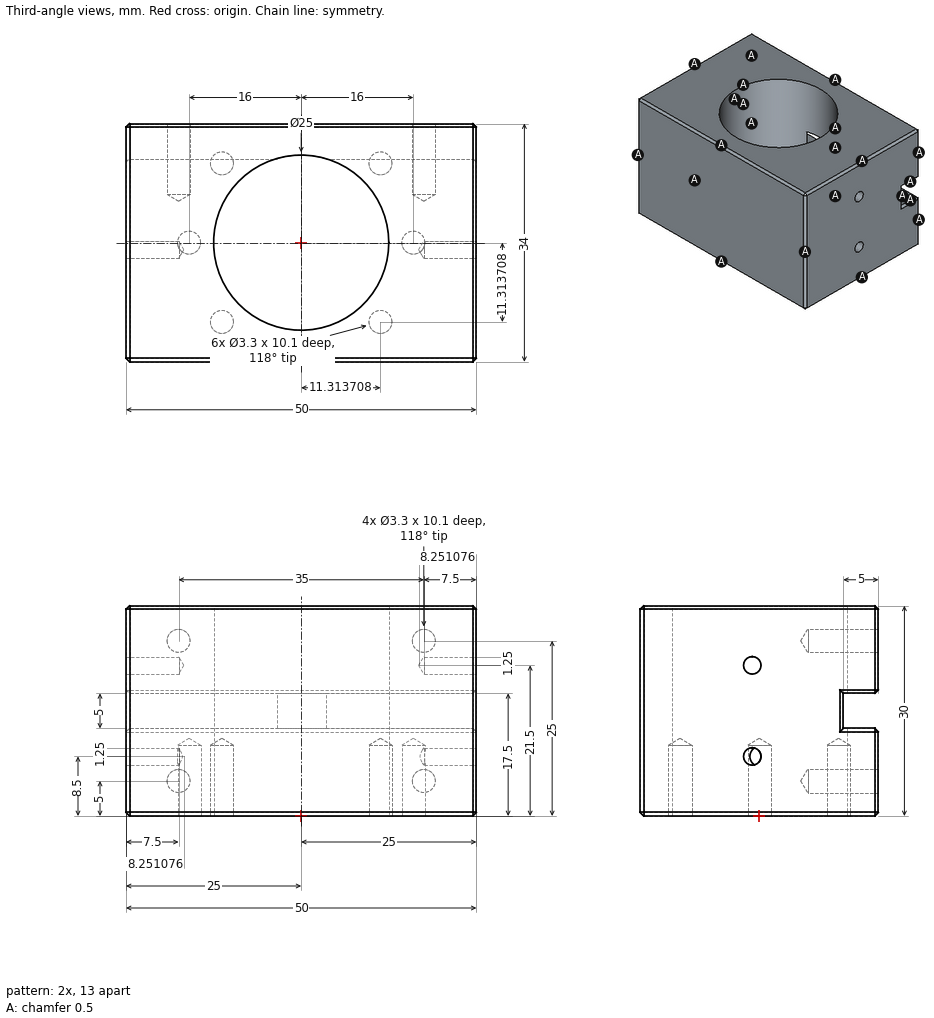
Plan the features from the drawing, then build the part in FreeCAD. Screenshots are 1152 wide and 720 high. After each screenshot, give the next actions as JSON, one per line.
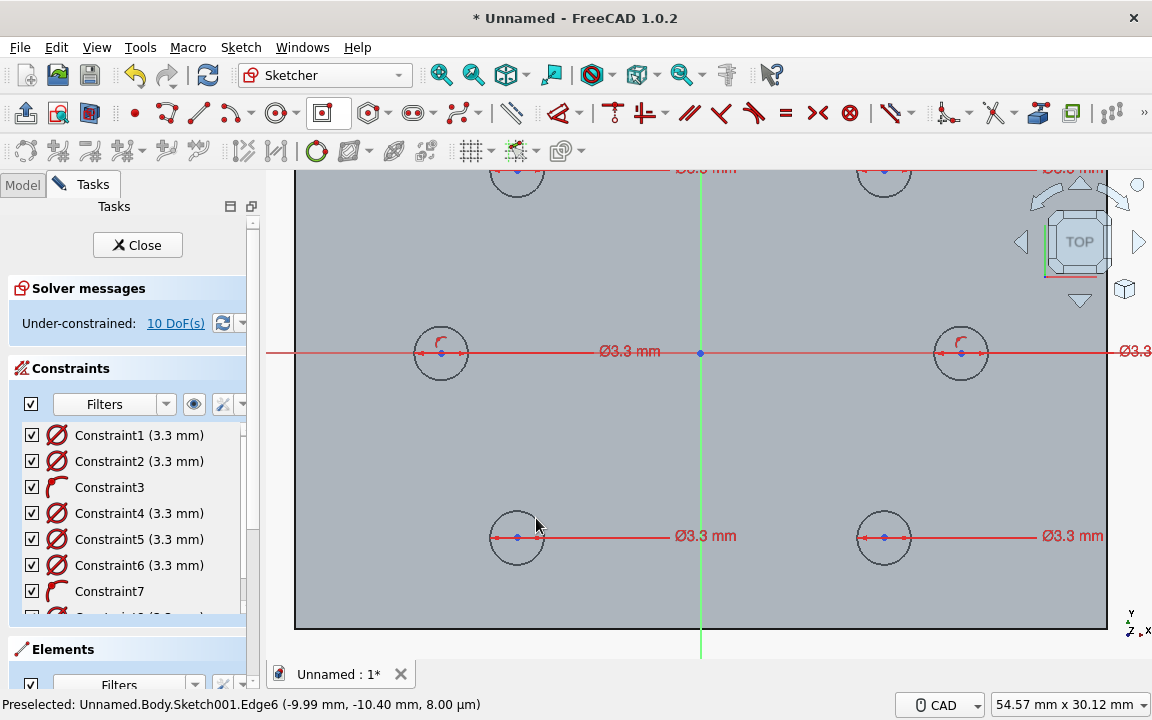
{"action": "left_click", "coordinate": [884, 538]}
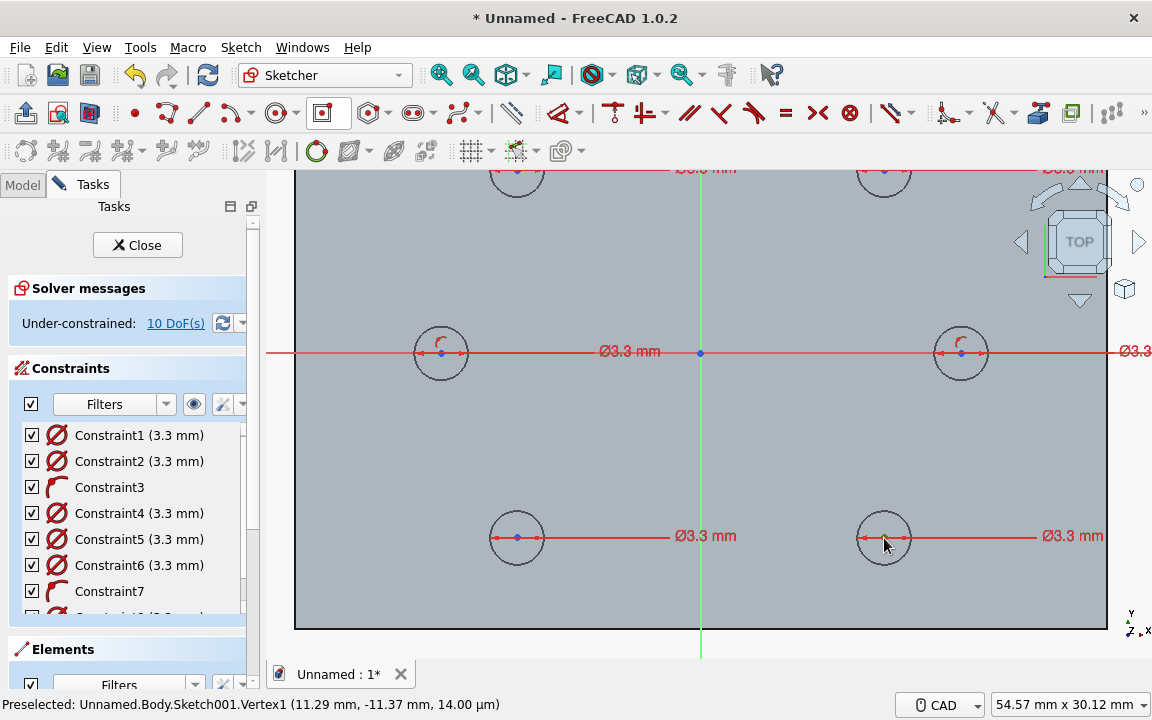
{"action": "scroll", "coordinate": [518, 539], "scroll_direction": "down", "scroll_amount": 2}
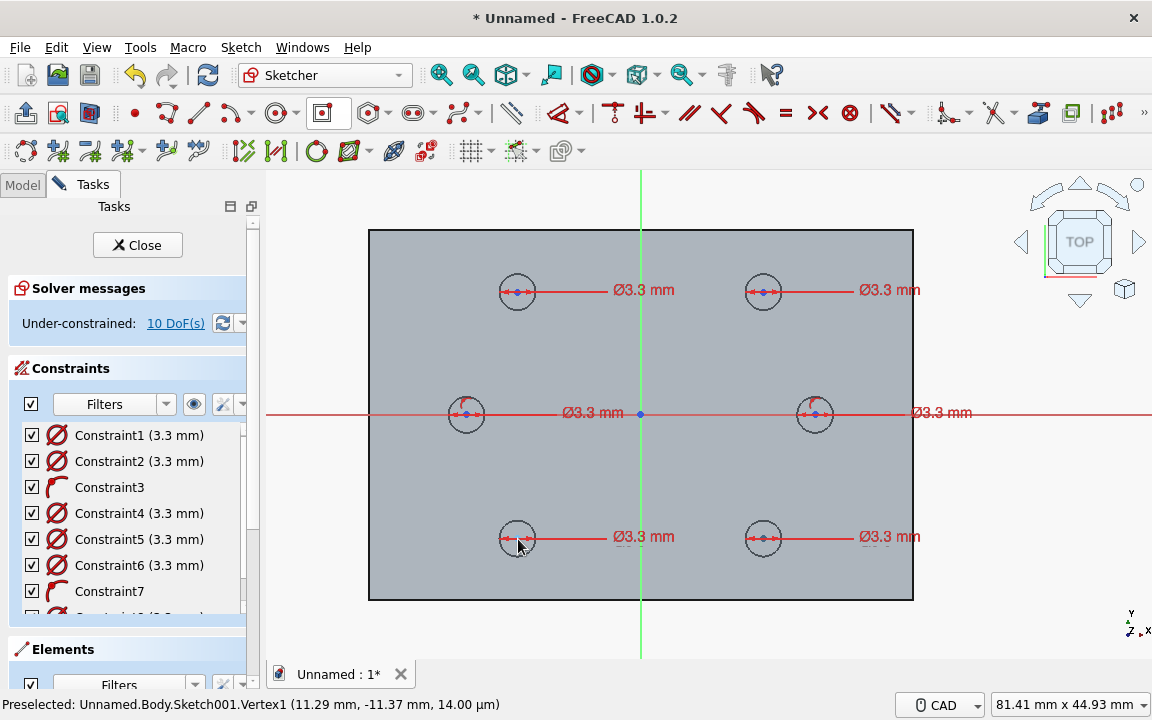
{"action": "left_click", "coordinate": [764, 292]}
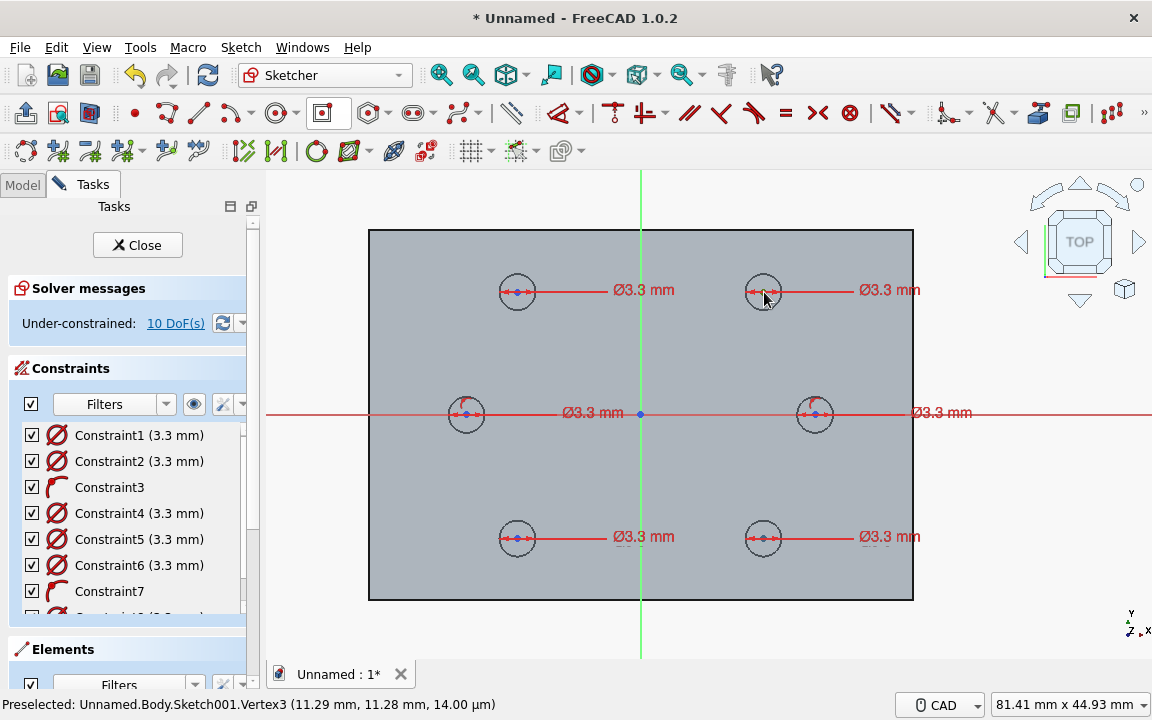
{"action": "left_click", "coordinate": [344, 415]}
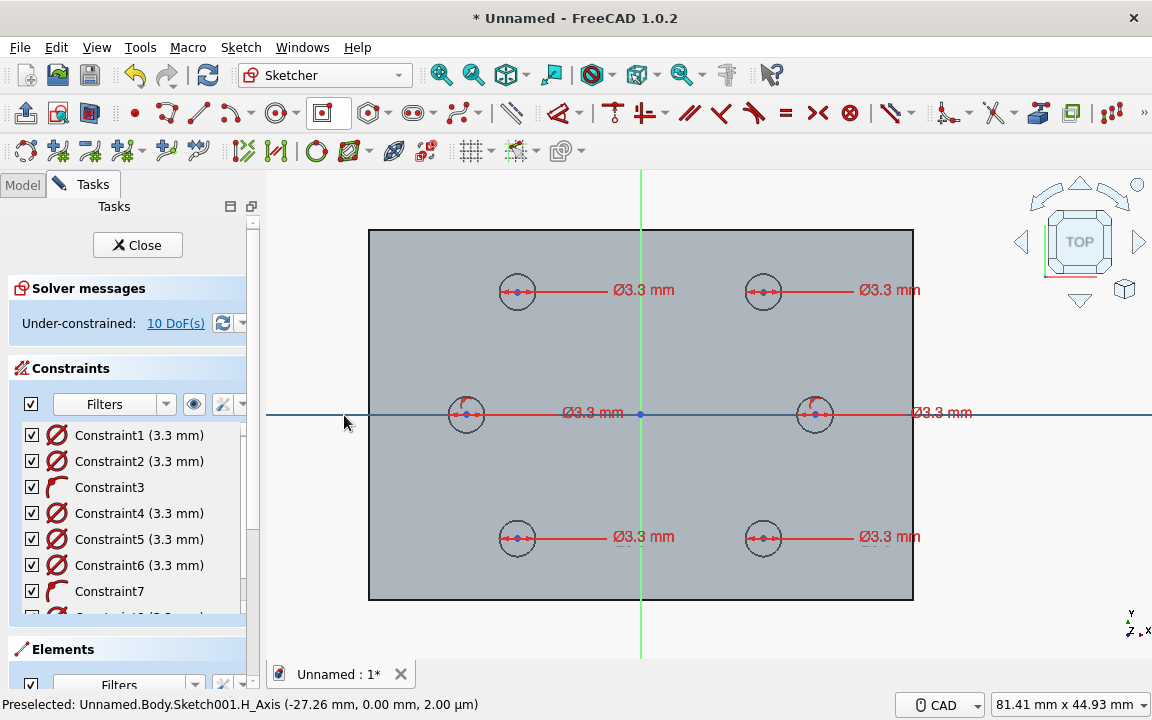
{"action": "key", "text": "s"}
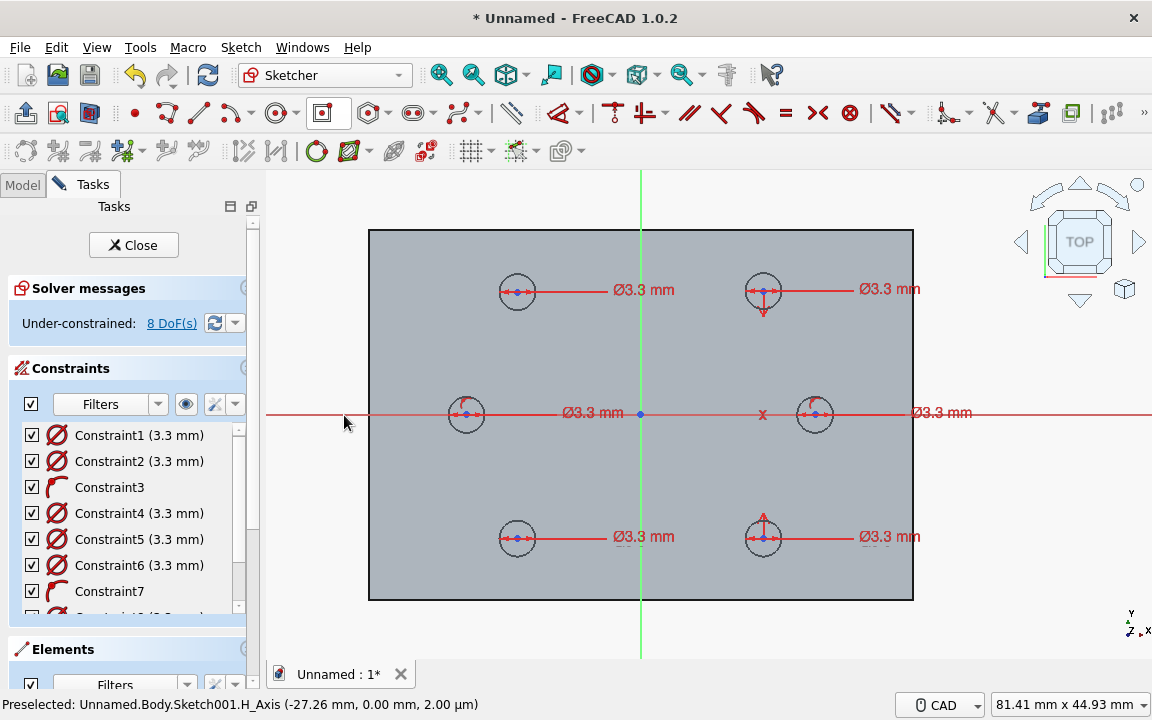
{"action": "left_click", "coordinate": [764, 291]}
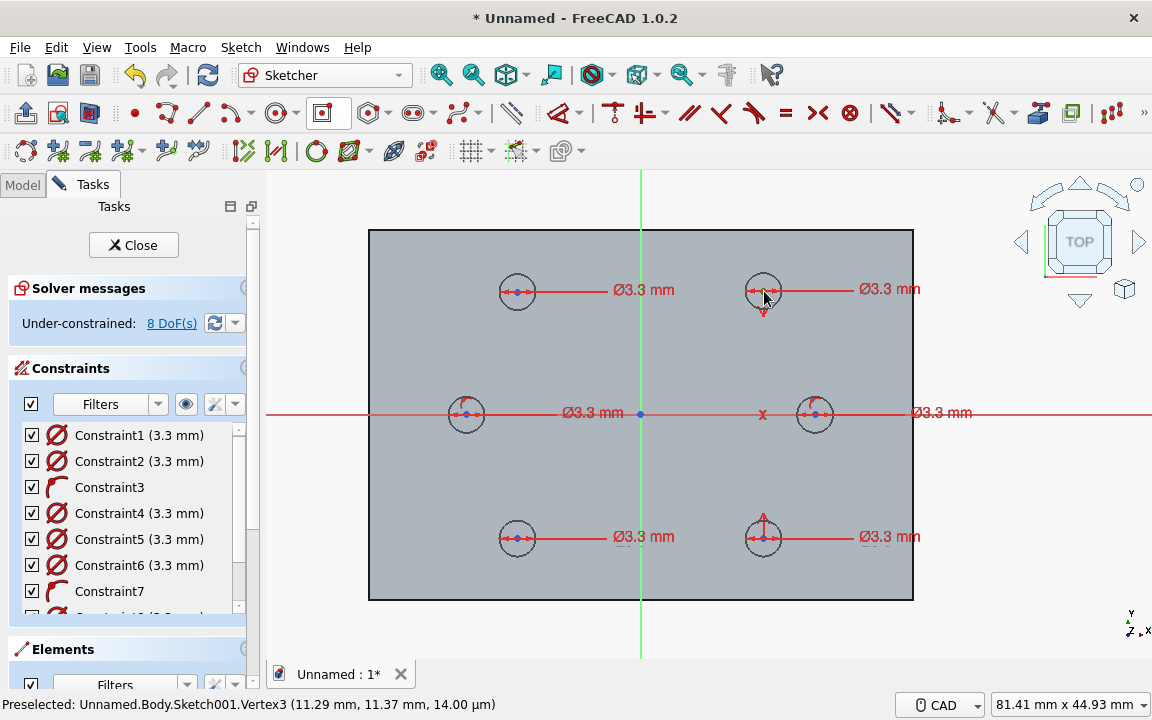
{"action": "left_click", "coordinate": [518, 292]}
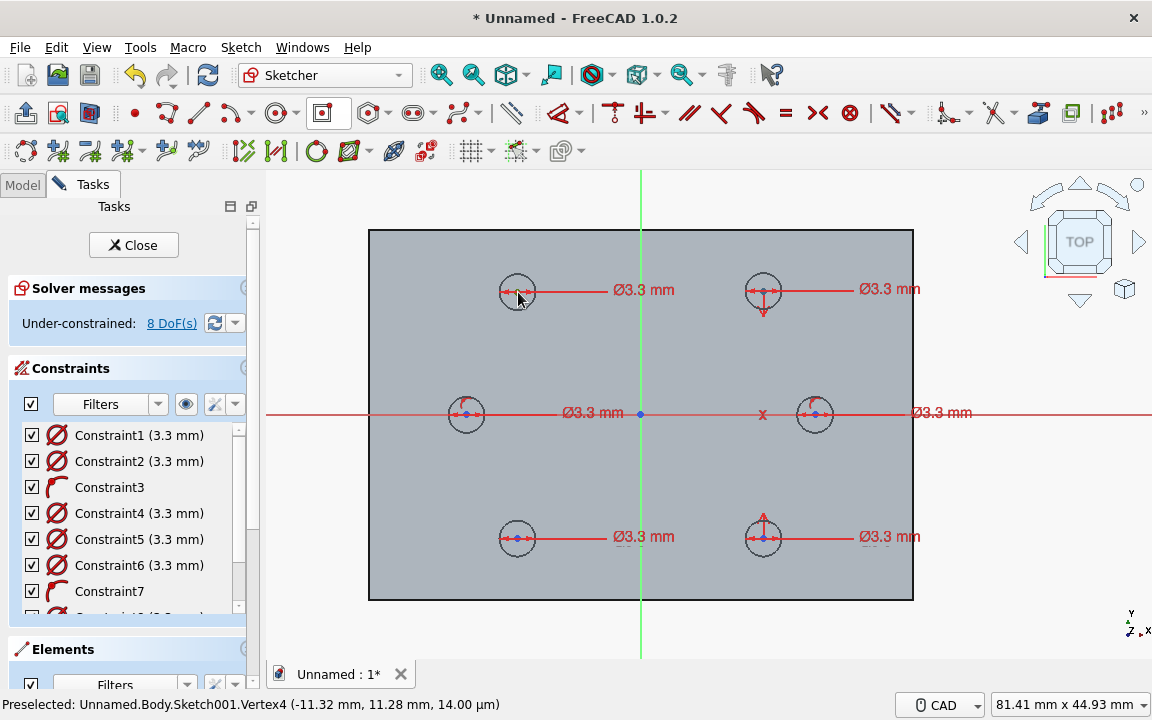
{"action": "left_click", "coordinate": [641, 600]}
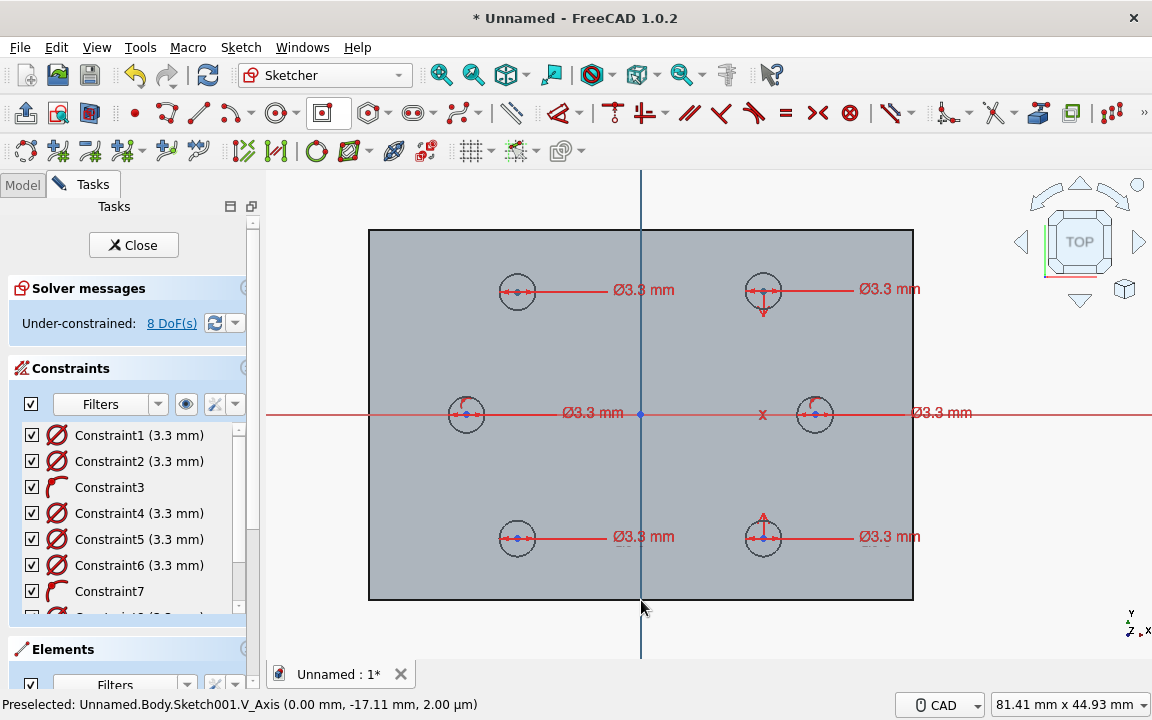
{"action": "key", "text": "s"}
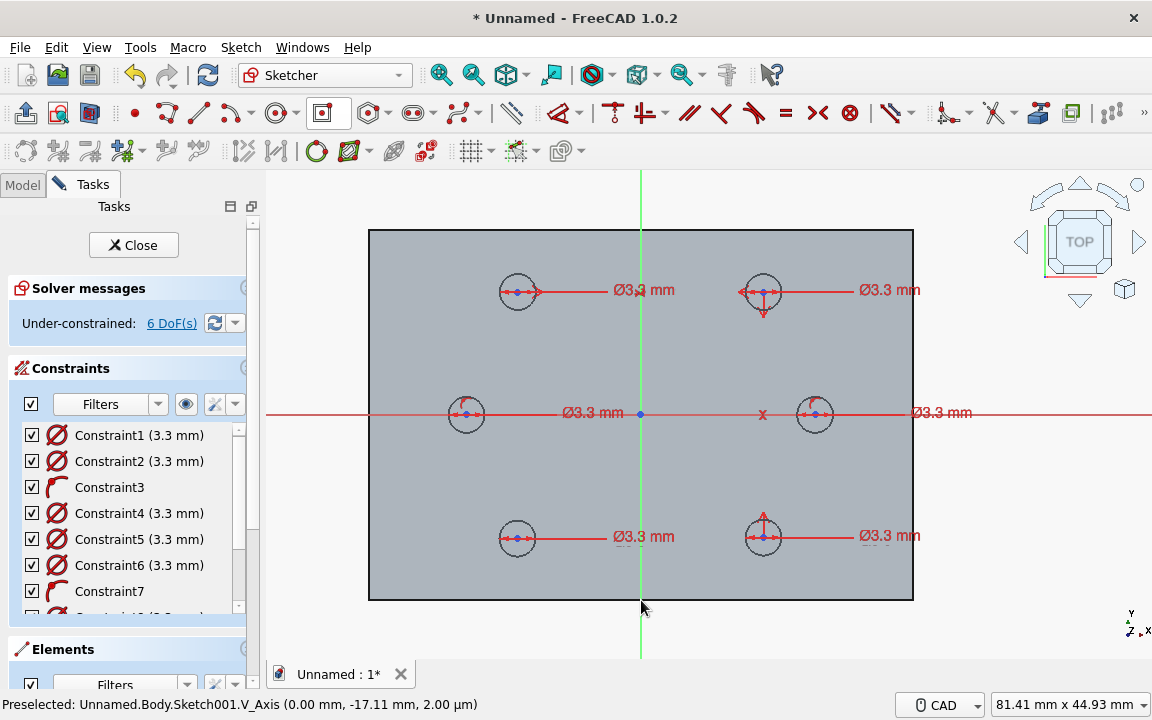
{"action": "left_click", "coordinate": [764, 538]}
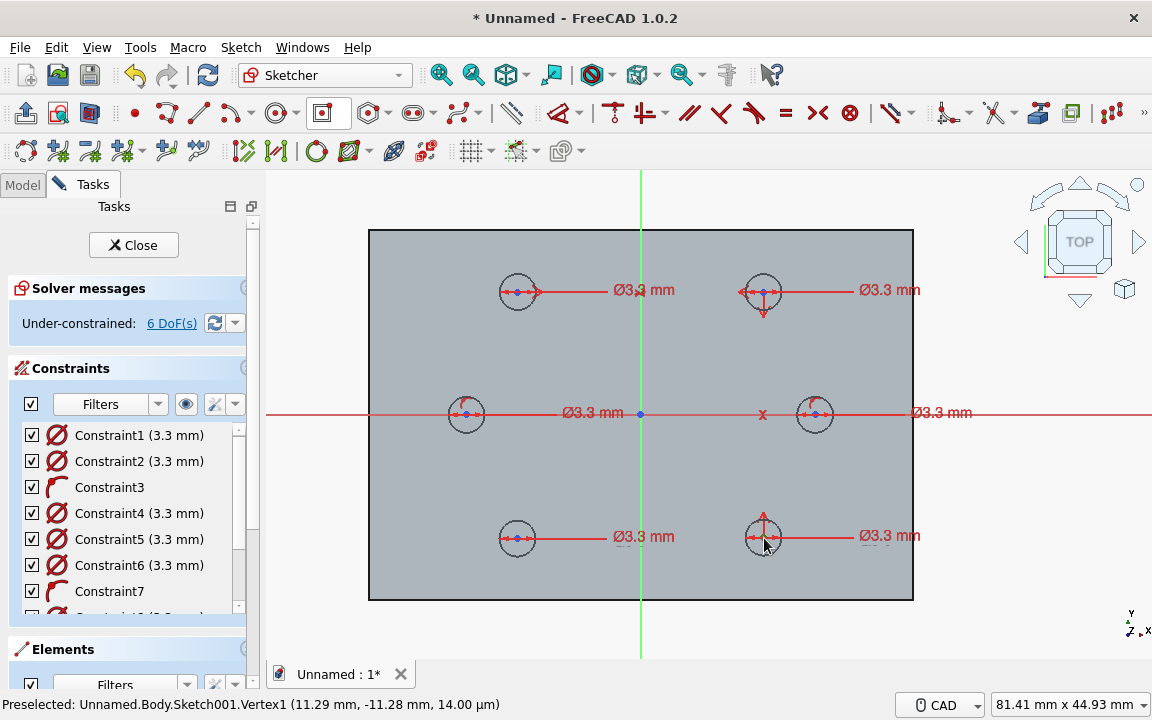
{"action": "left_click", "coordinate": [517, 539]}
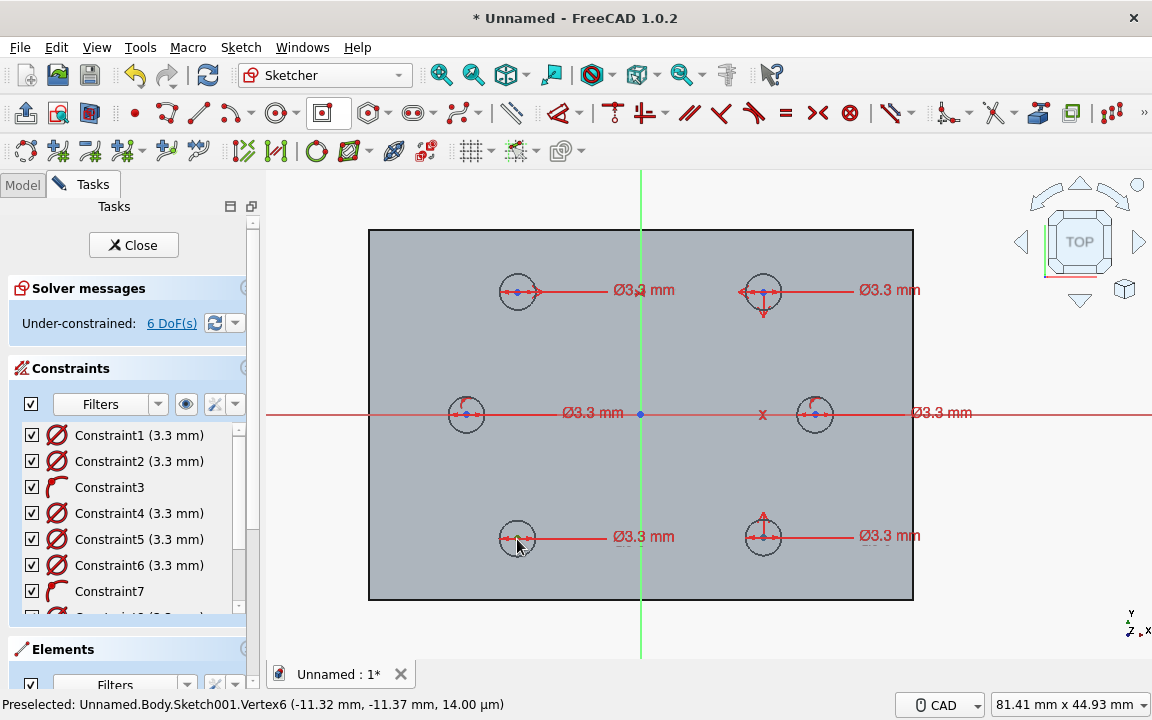
{"action": "left_click", "coordinate": [641, 600]}